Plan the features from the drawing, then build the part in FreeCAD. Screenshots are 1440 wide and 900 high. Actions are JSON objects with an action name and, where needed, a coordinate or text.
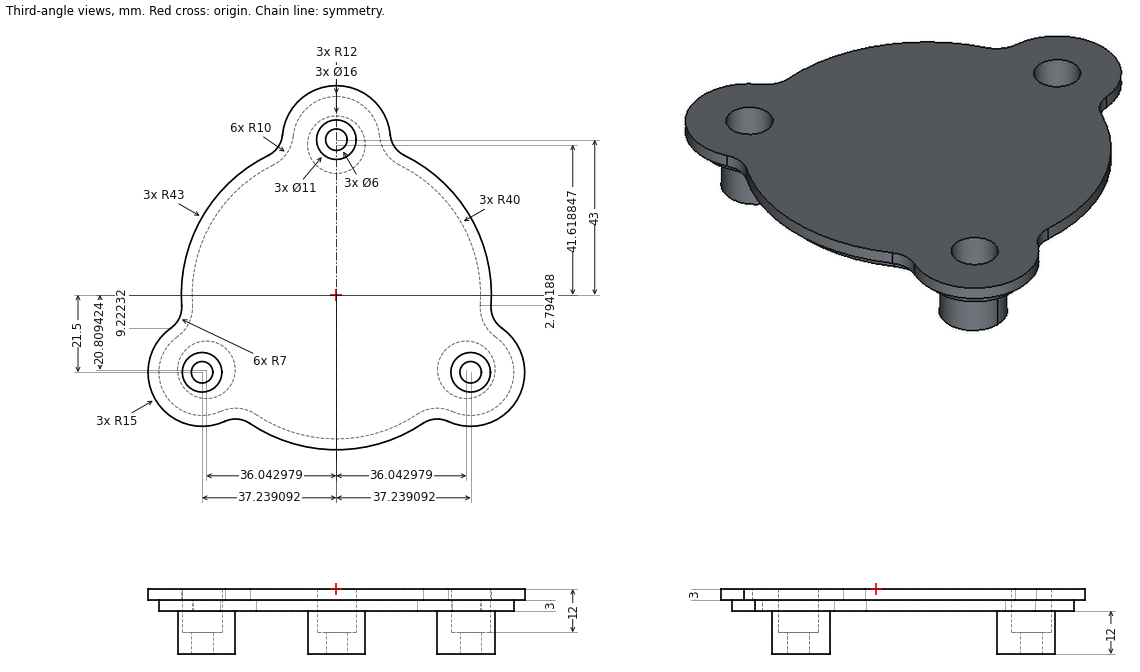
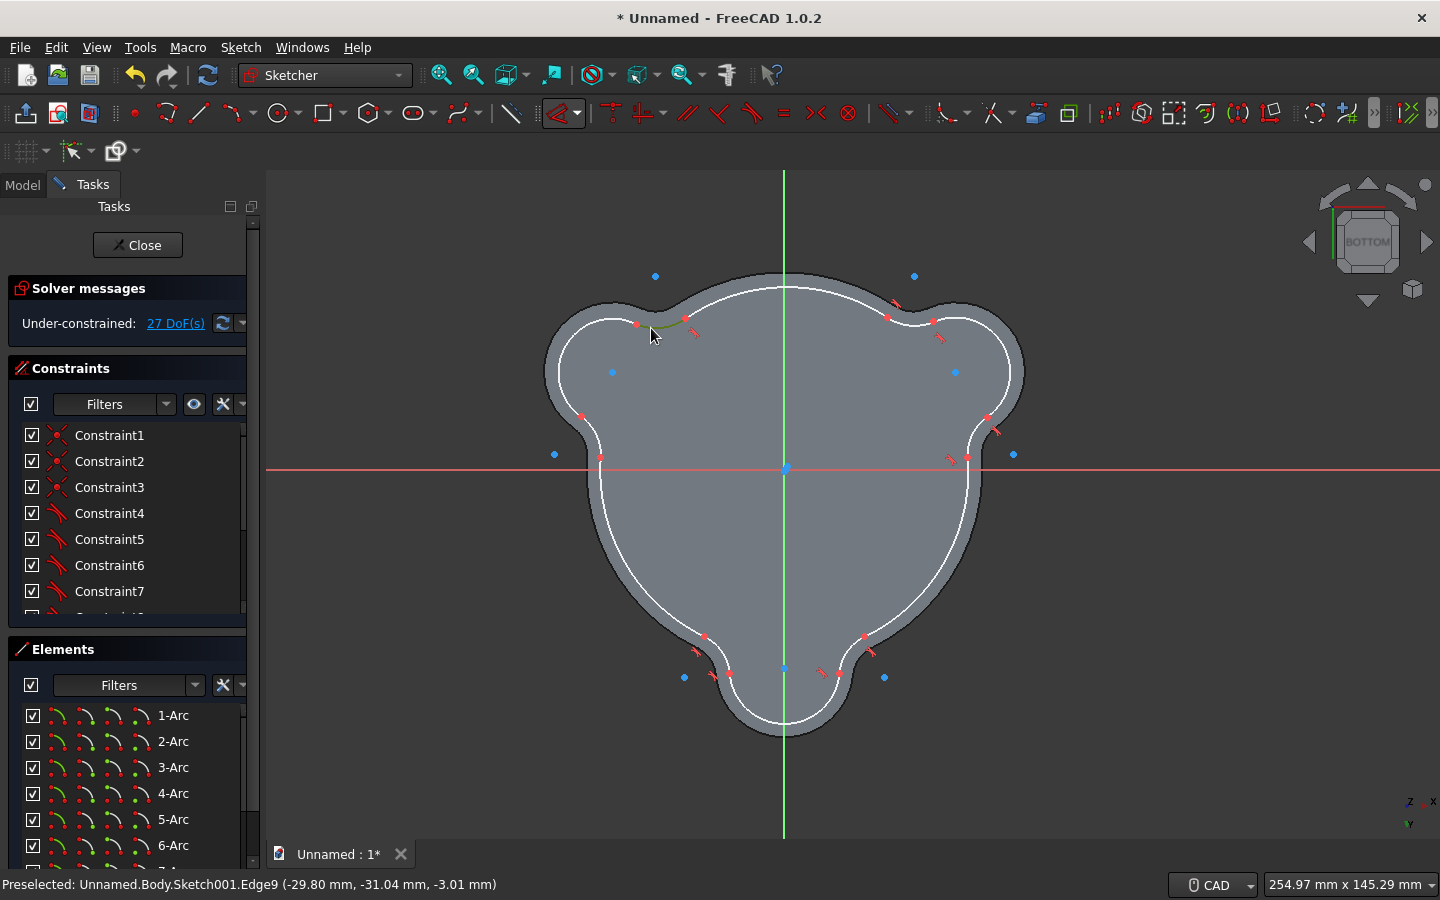
{"action": "left_click", "coordinate": [590, 324]}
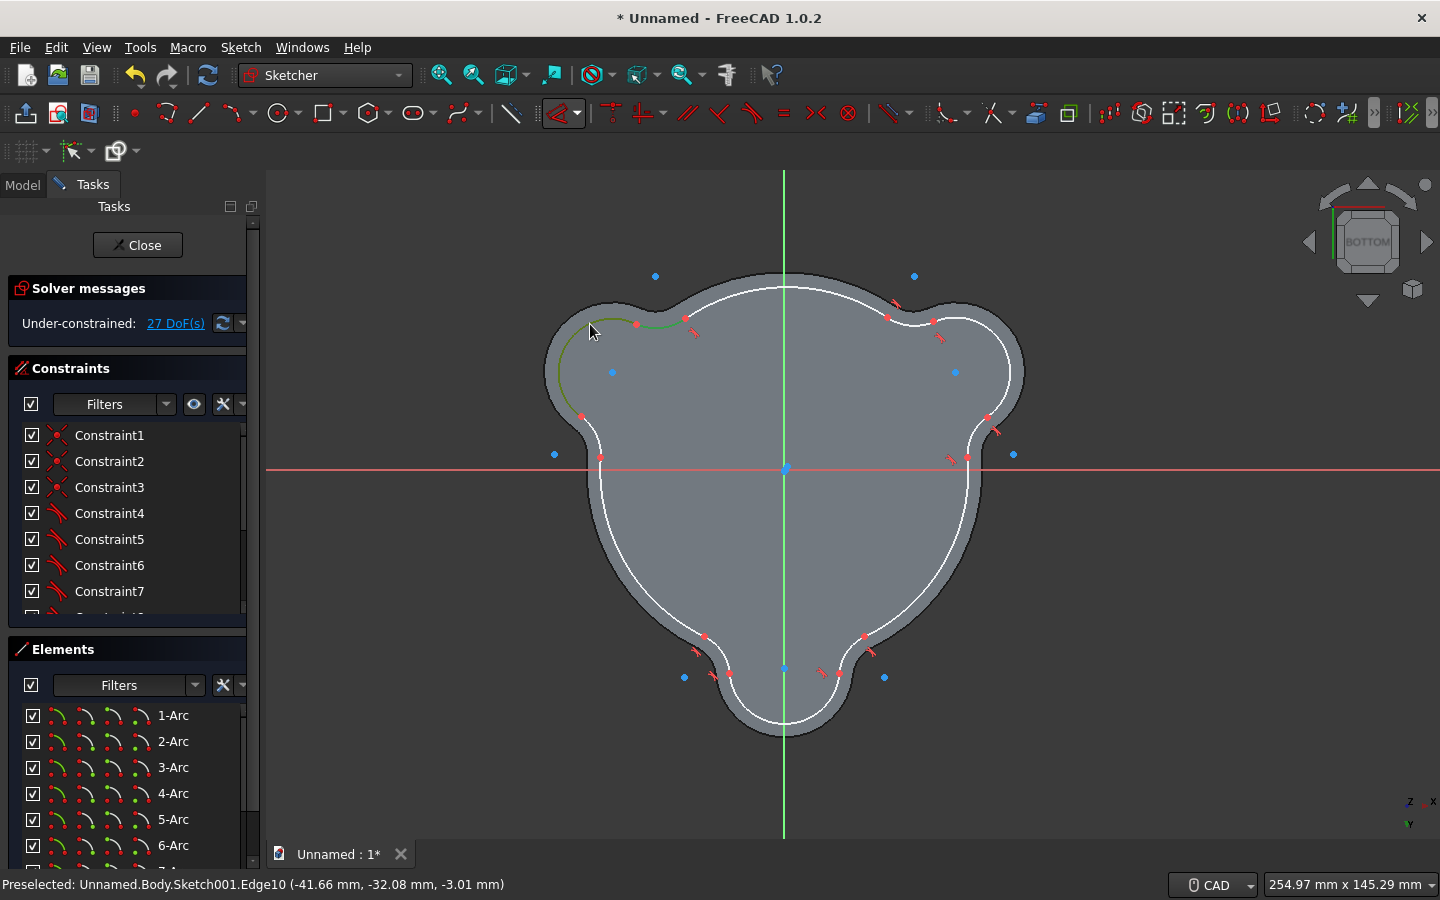
{"action": "left_click", "coordinate": [752, 114]}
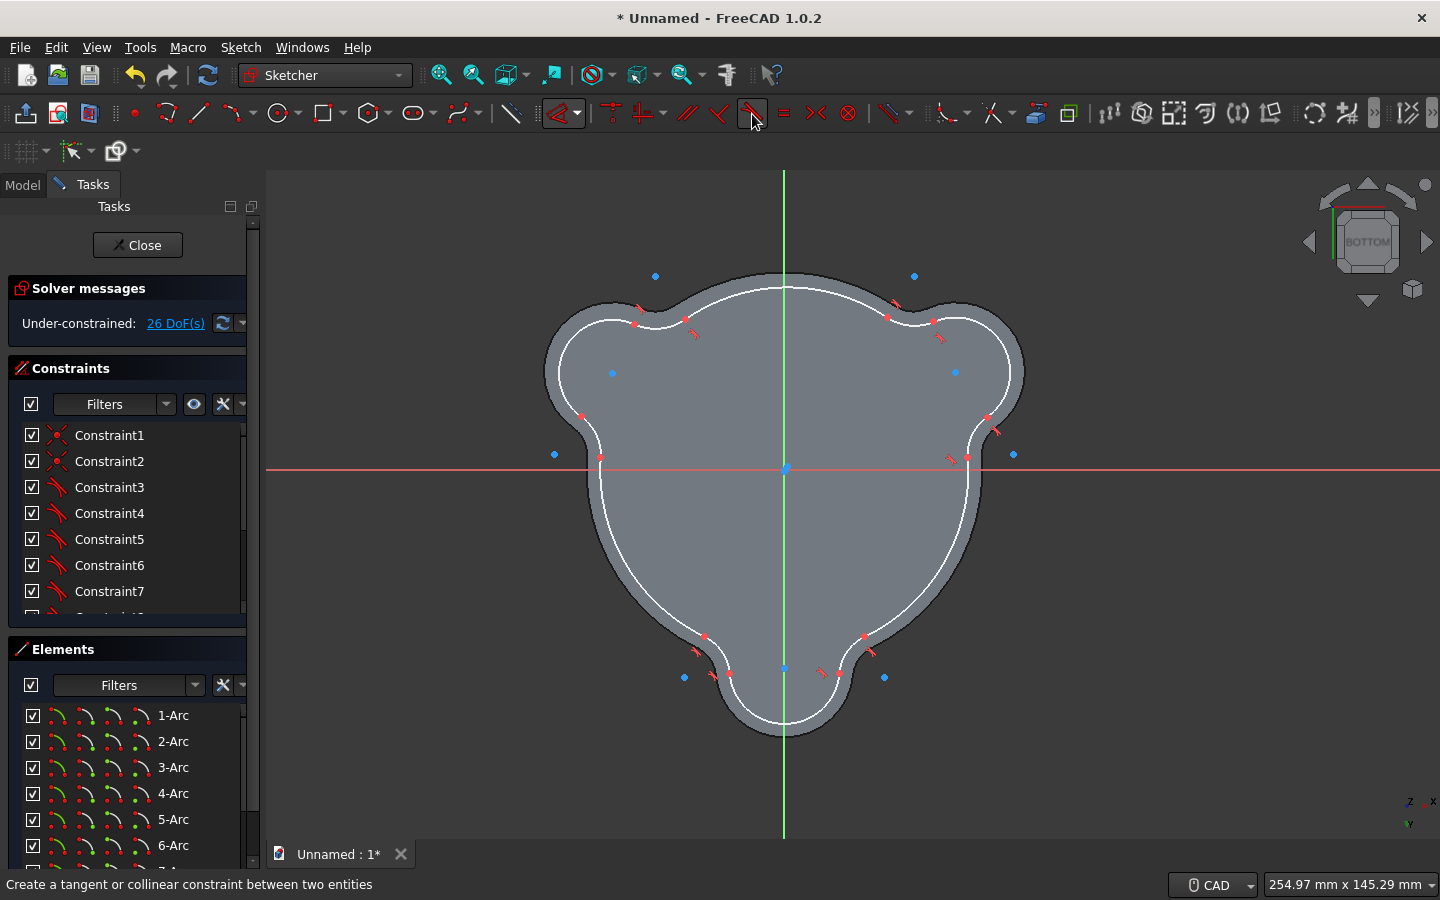
{"action": "left_click", "coordinate": [589, 325]}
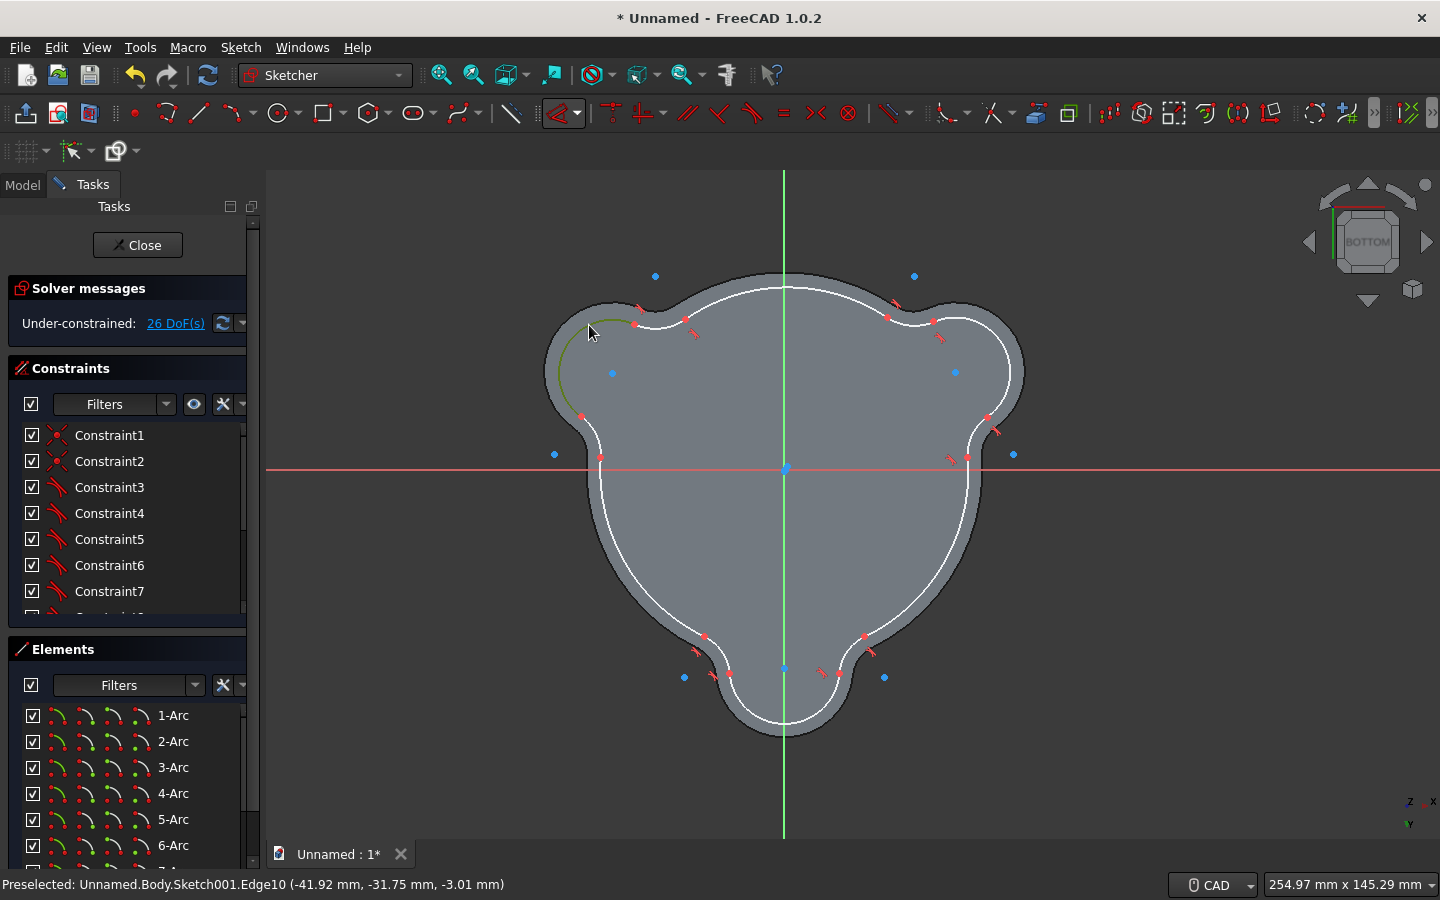
{"action": "left_click", "coordinate": [599, 444]}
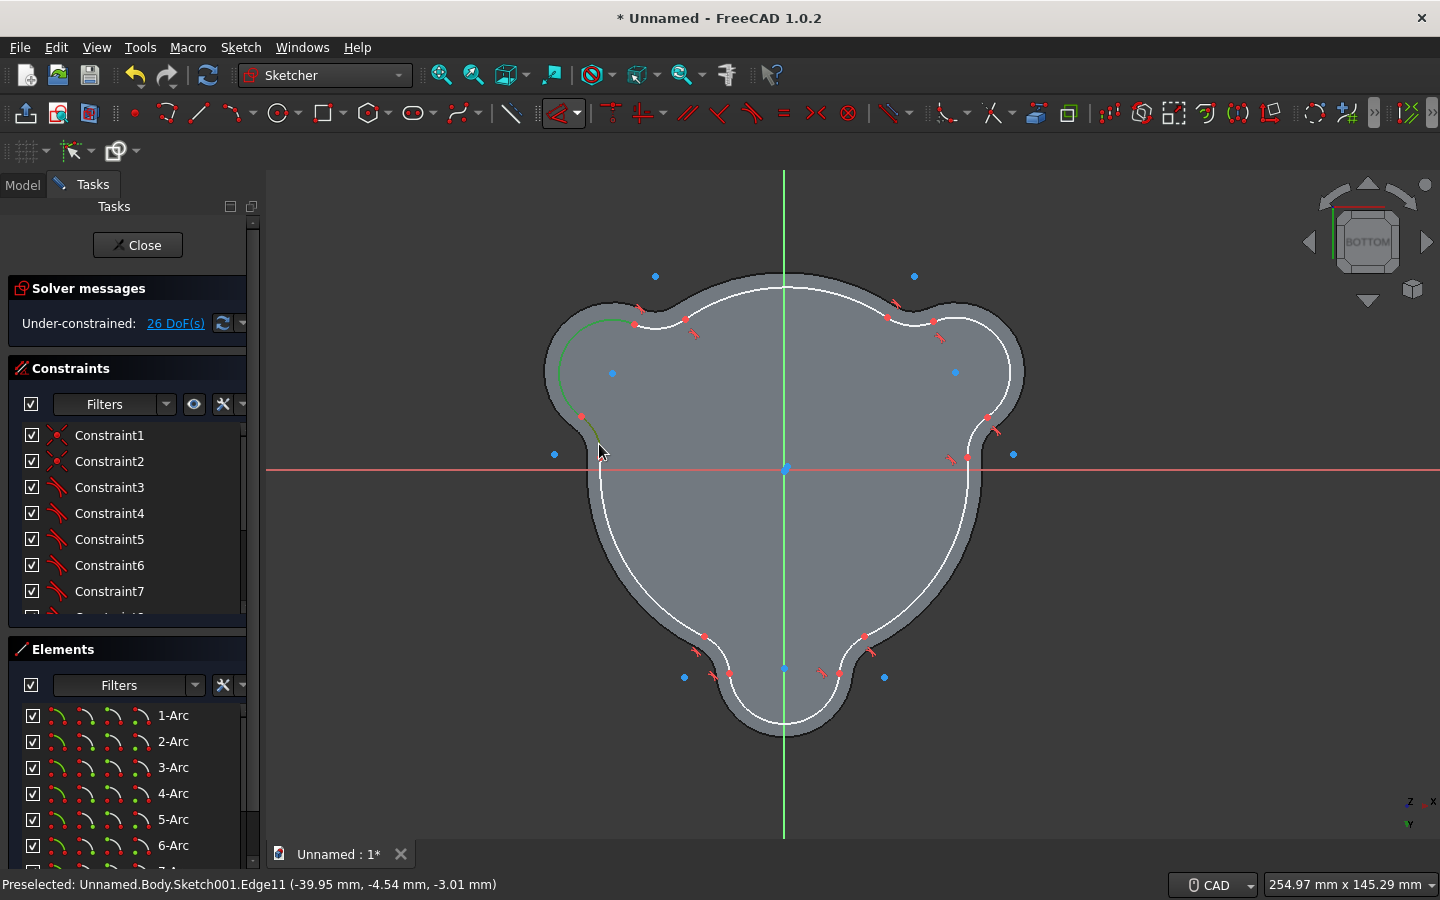
{"action": "left_click", "coordinate": [752, 114]}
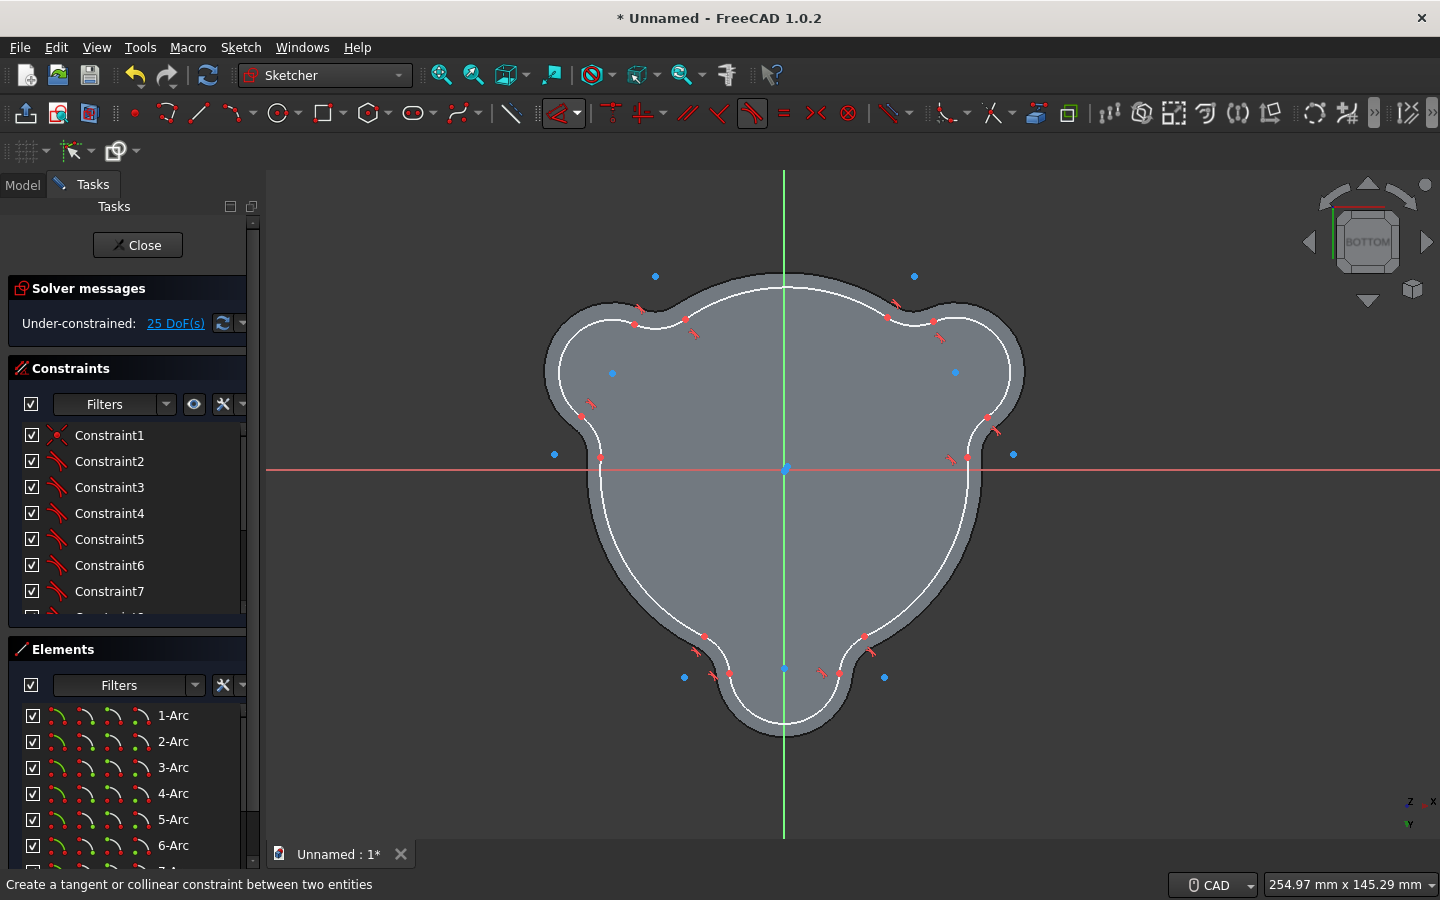
{"action": "left_click", "coordinate": [600, 444]}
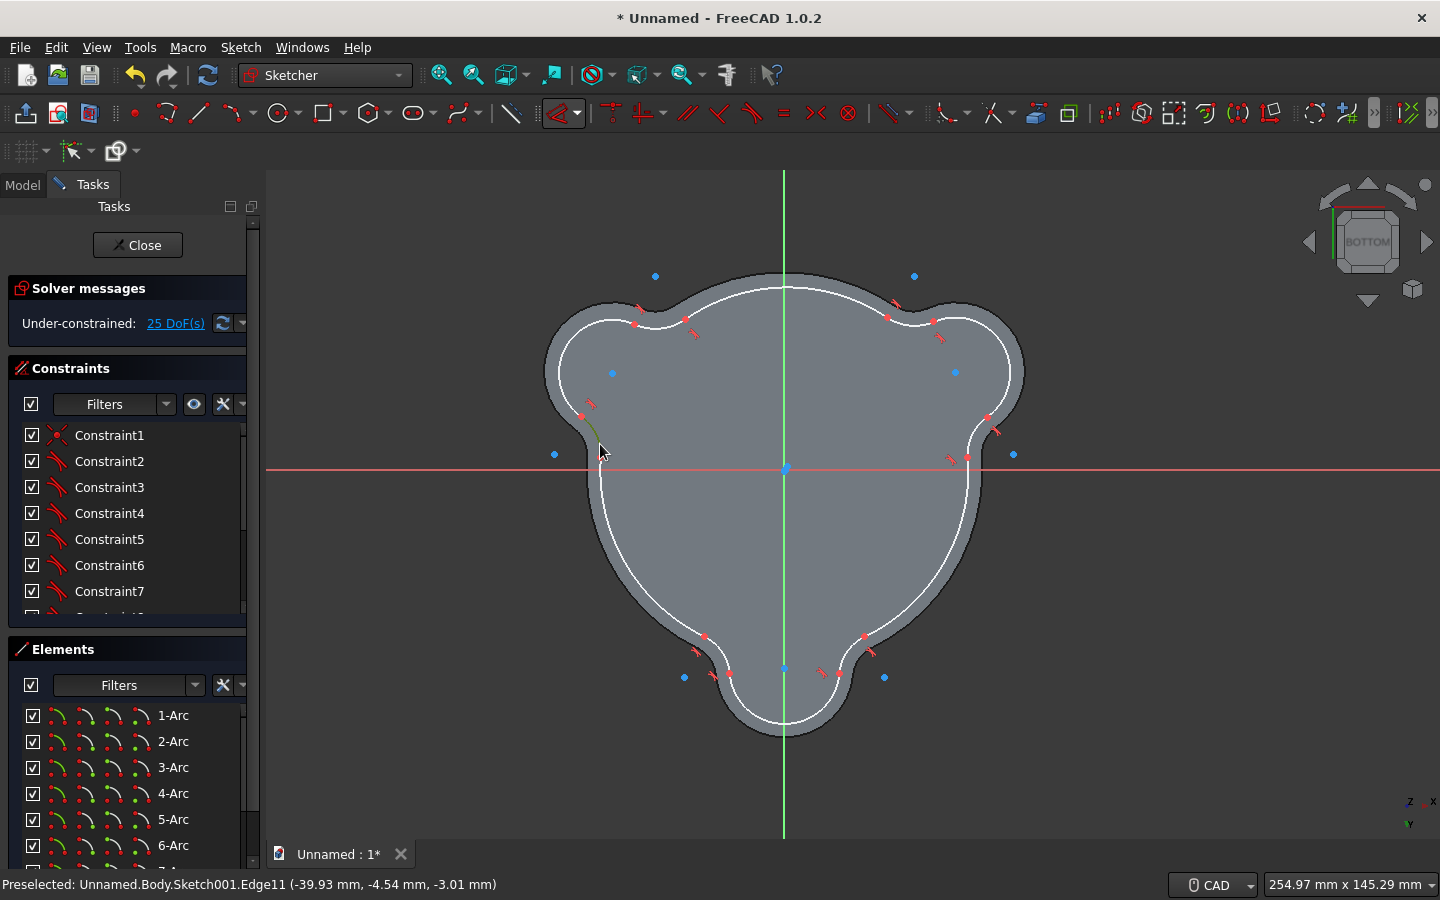
{"action": "left_click", "coordinate": [608, 523]}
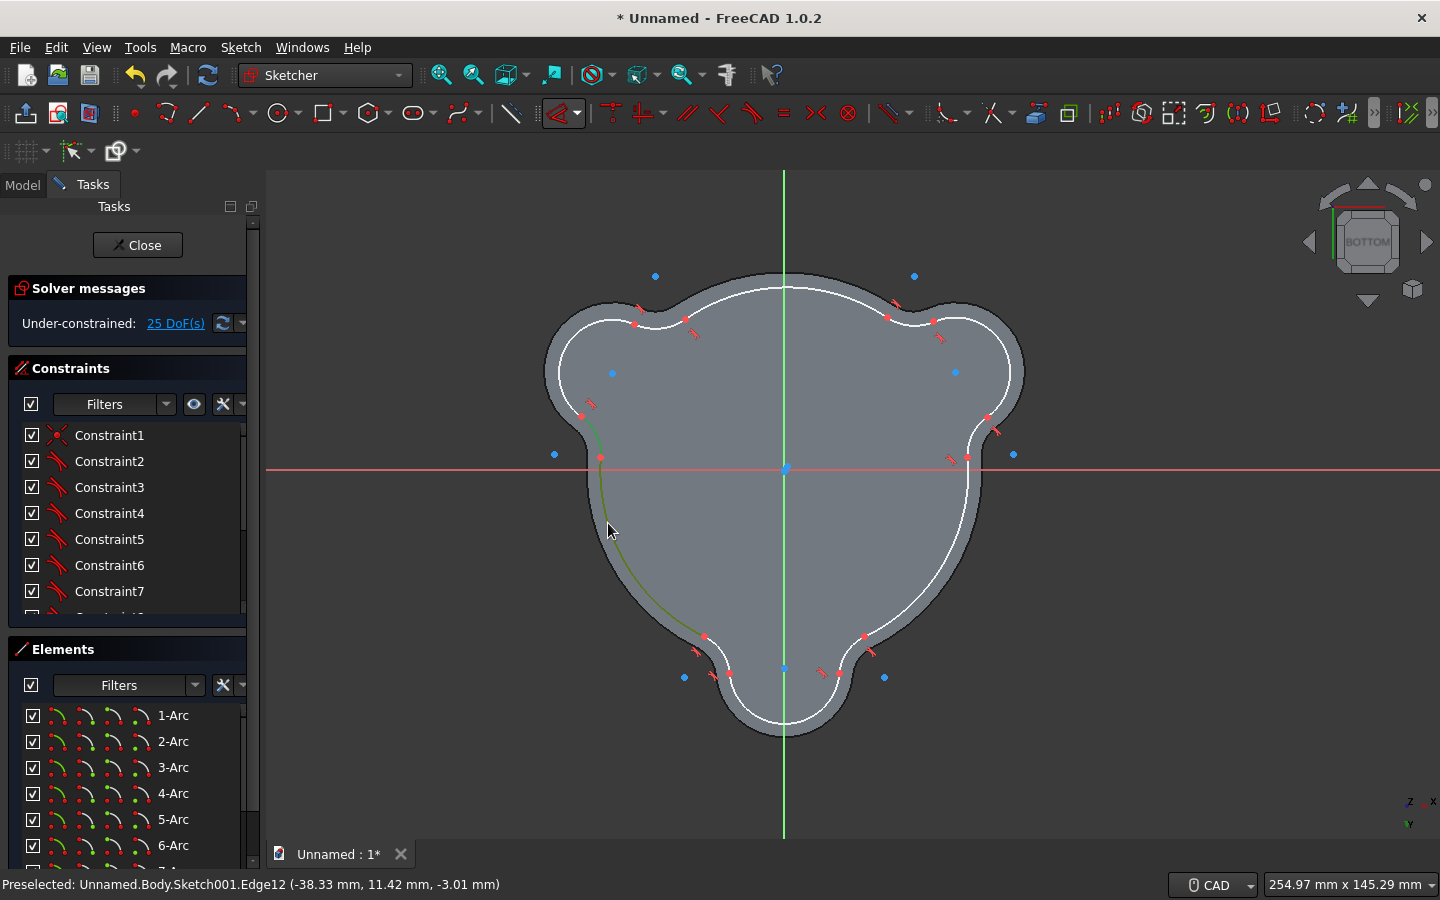
{"action": "left_click", "coordinate": [752, 114]}